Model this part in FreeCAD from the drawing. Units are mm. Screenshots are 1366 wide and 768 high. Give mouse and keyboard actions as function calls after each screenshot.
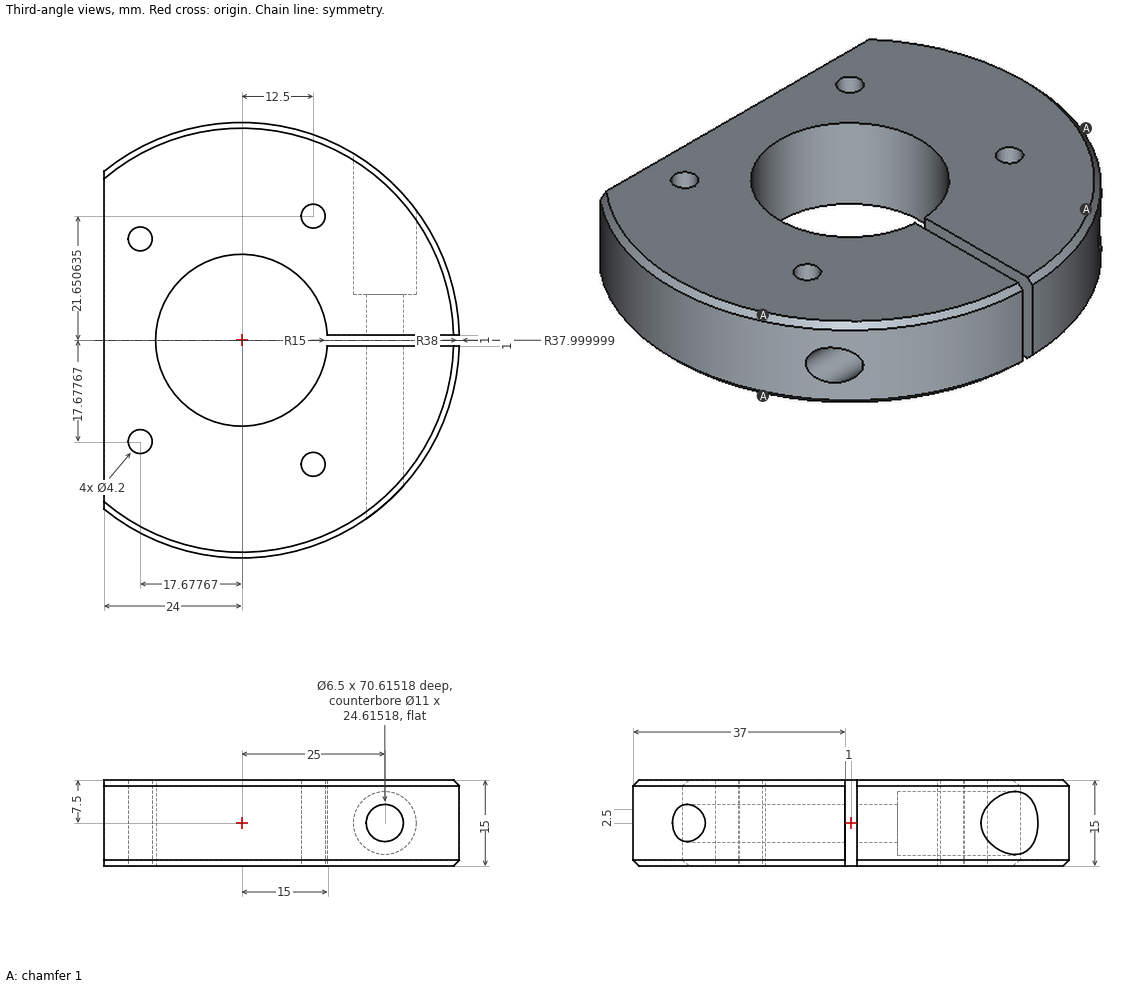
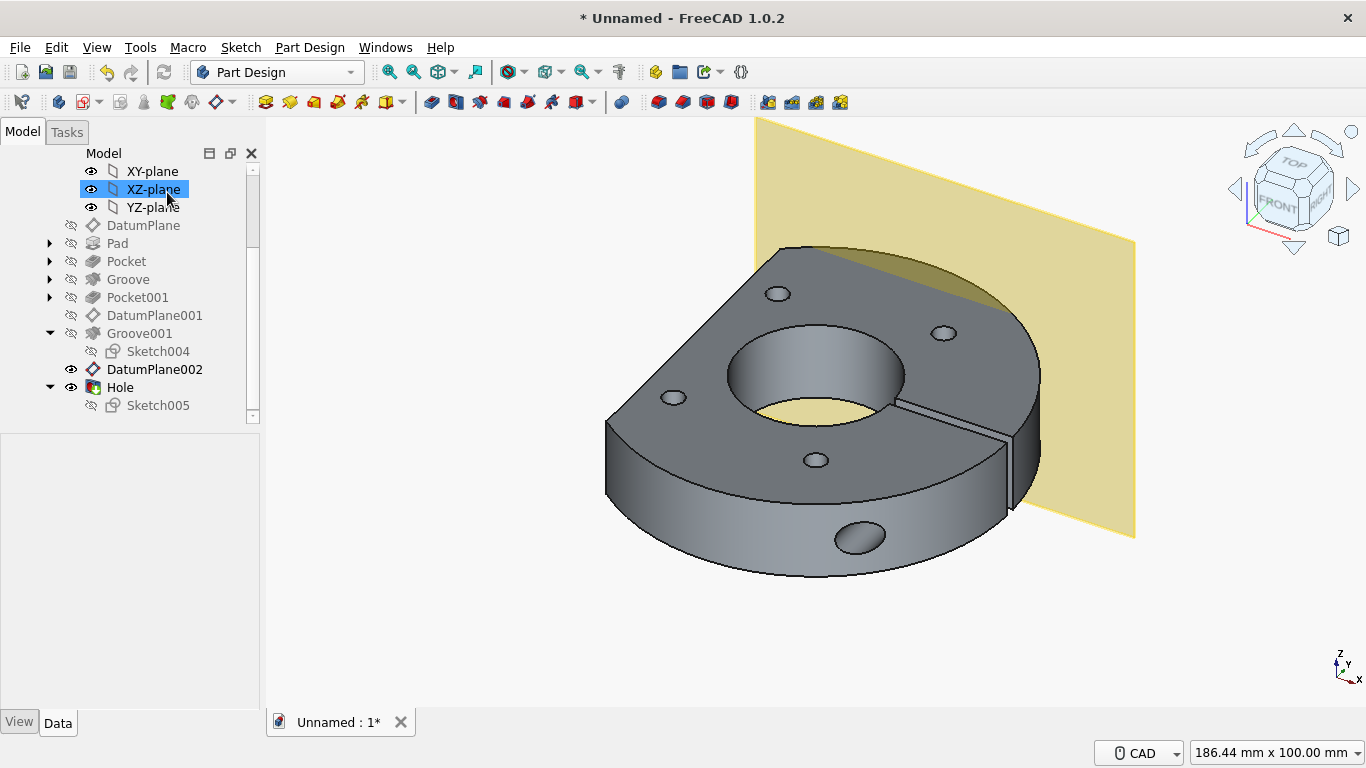
click(116, 369)
key(space)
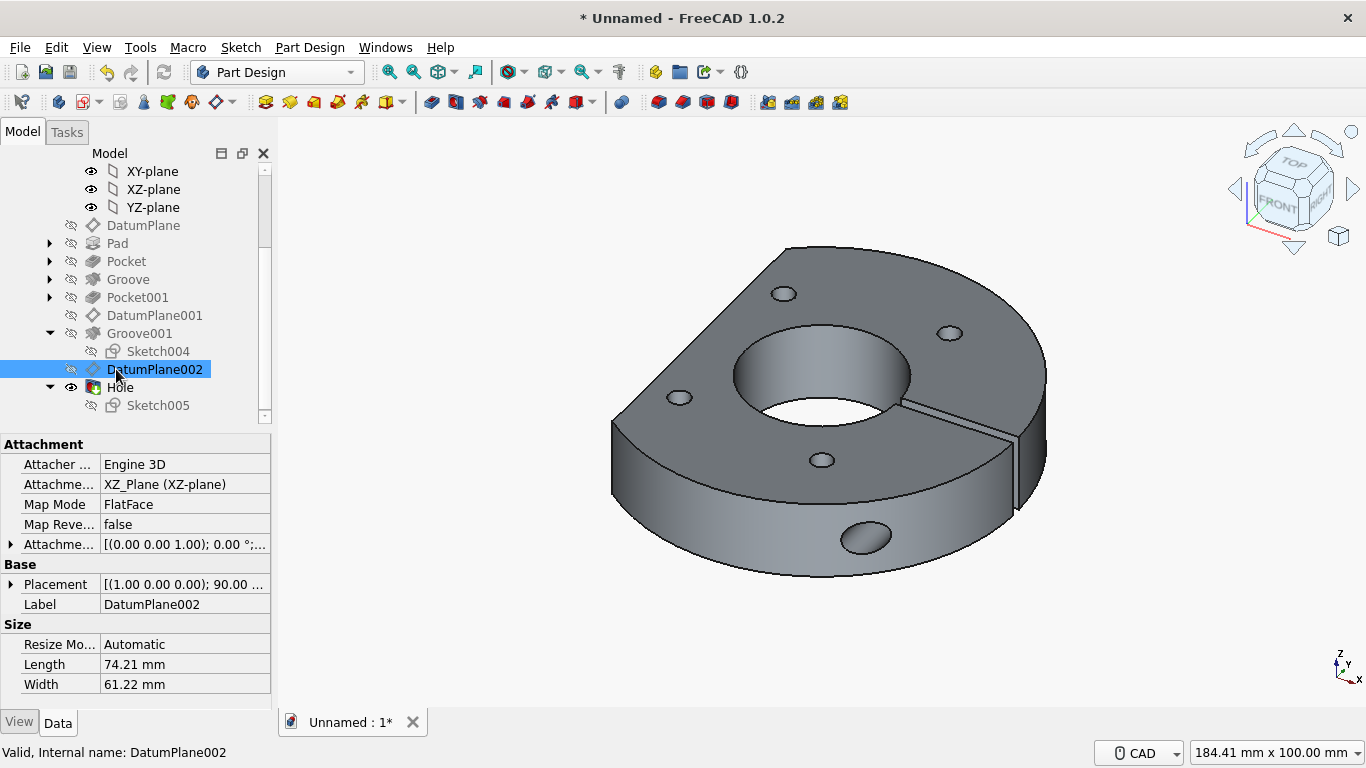
click(801, 503)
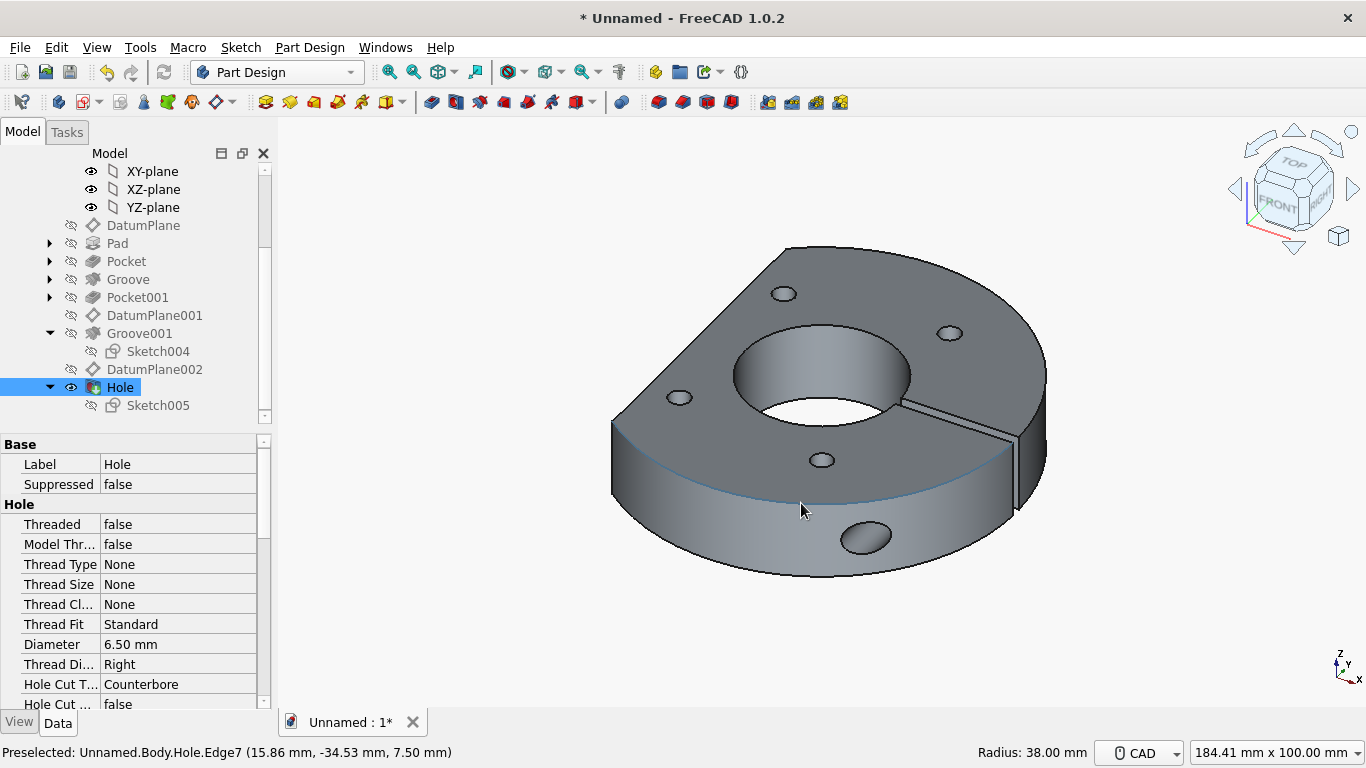
click(1046, 381, ctrl)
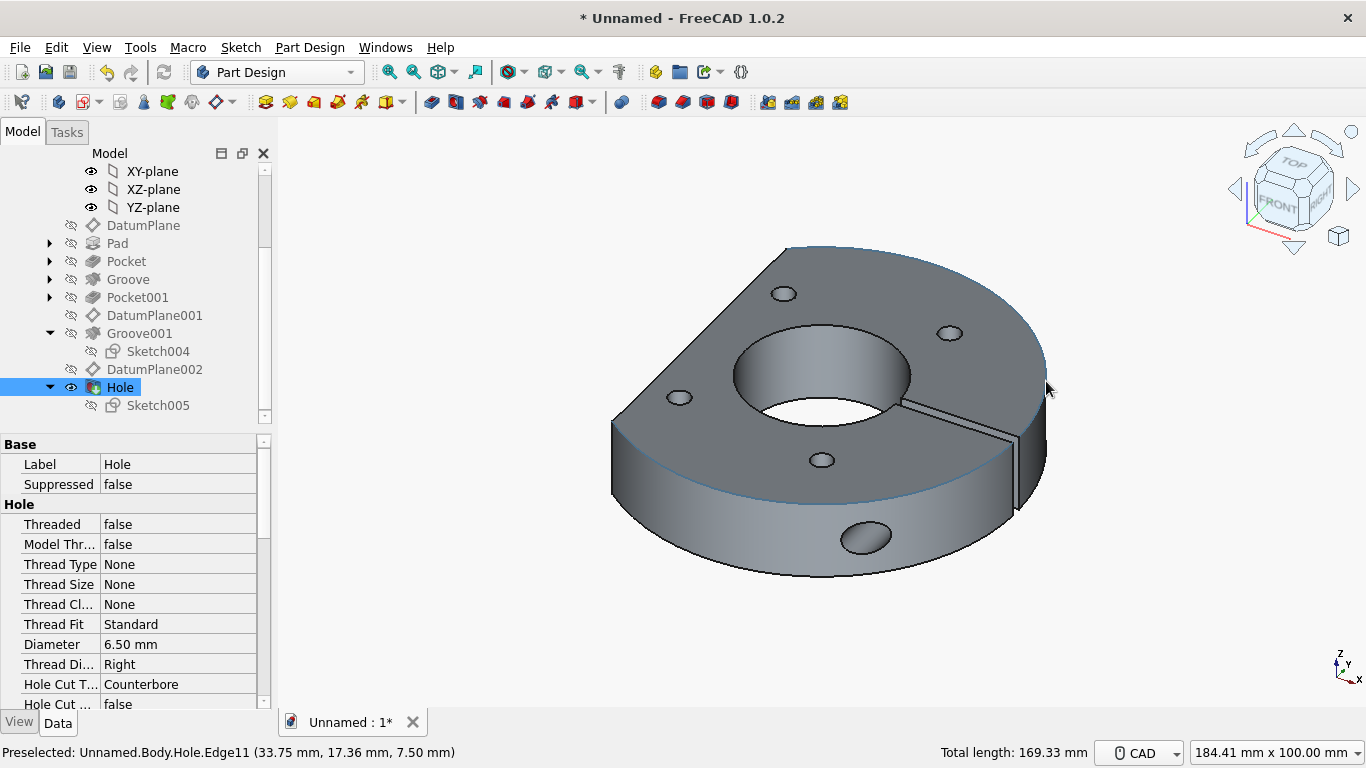
key(0)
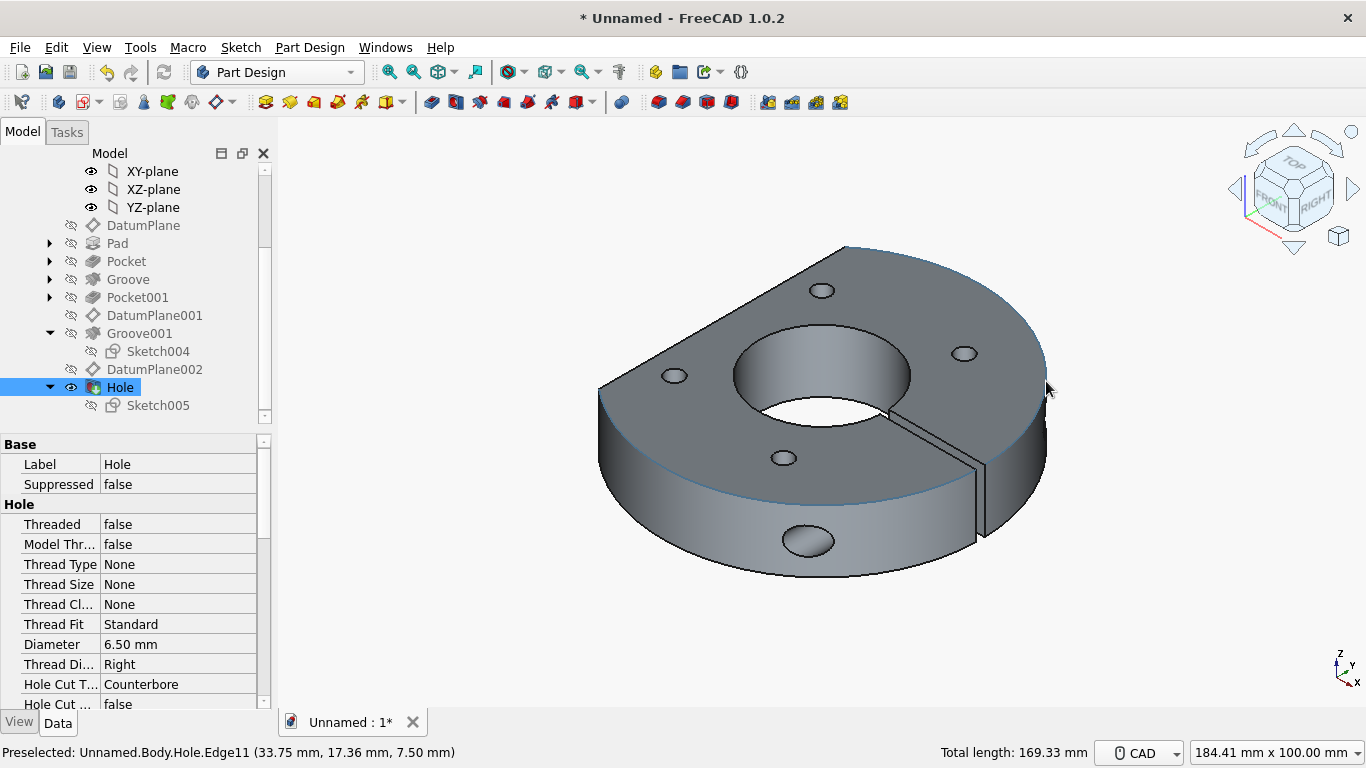
key(2)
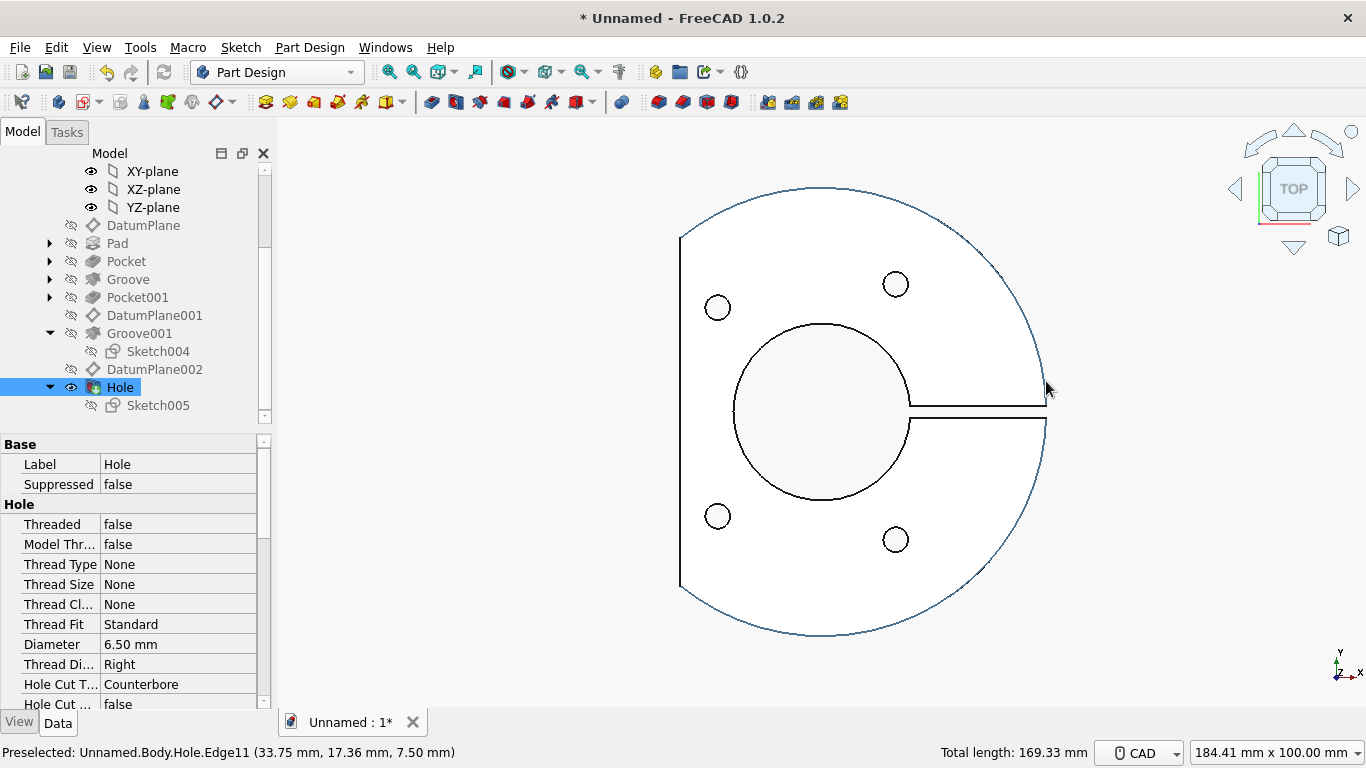
key(1)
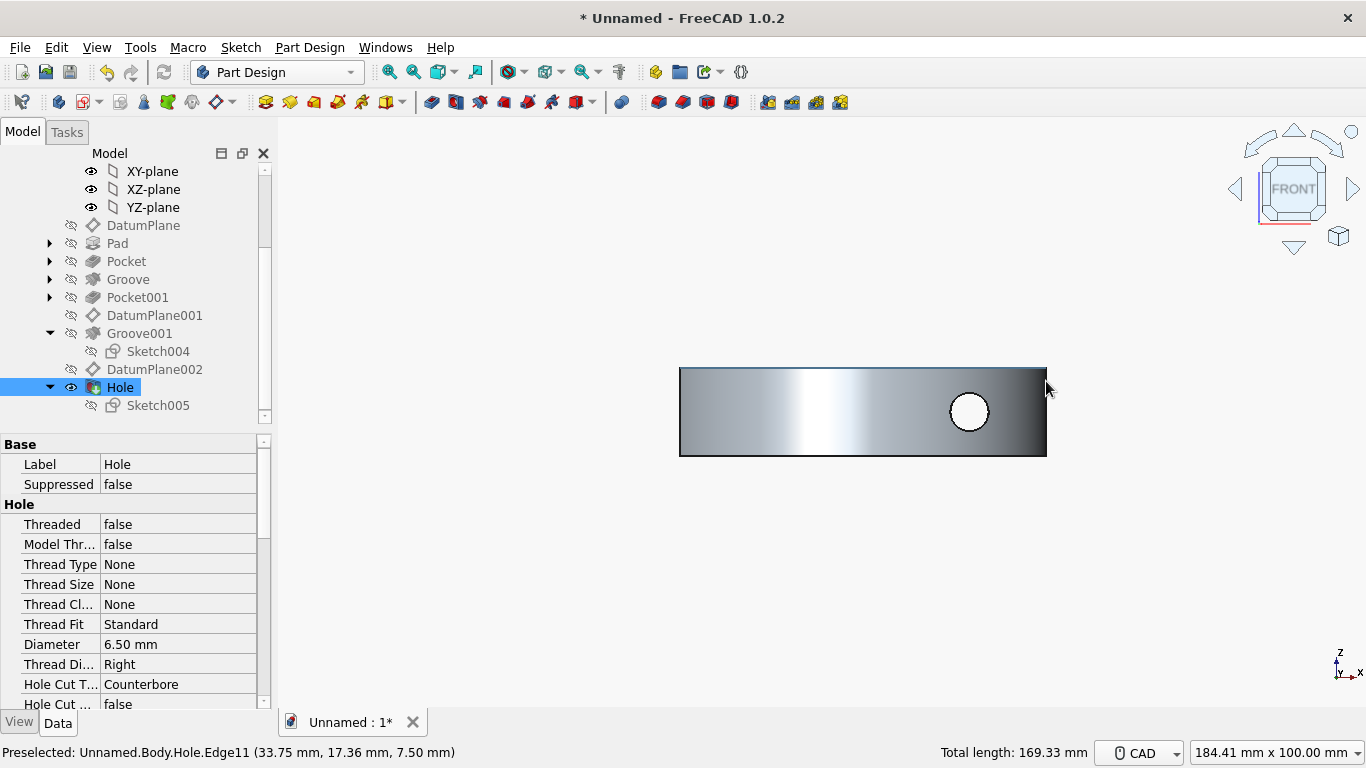
key(v)
key(f)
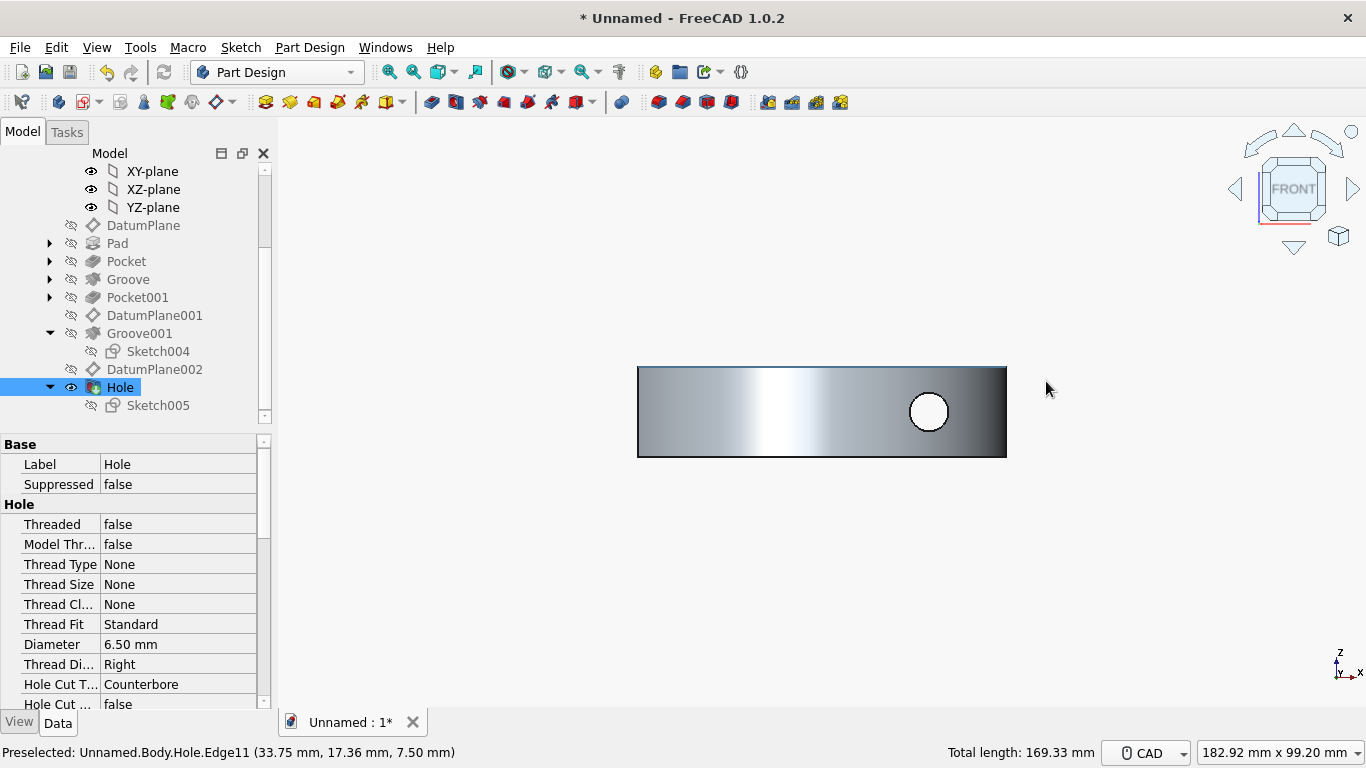
click(875, 456, ctrl)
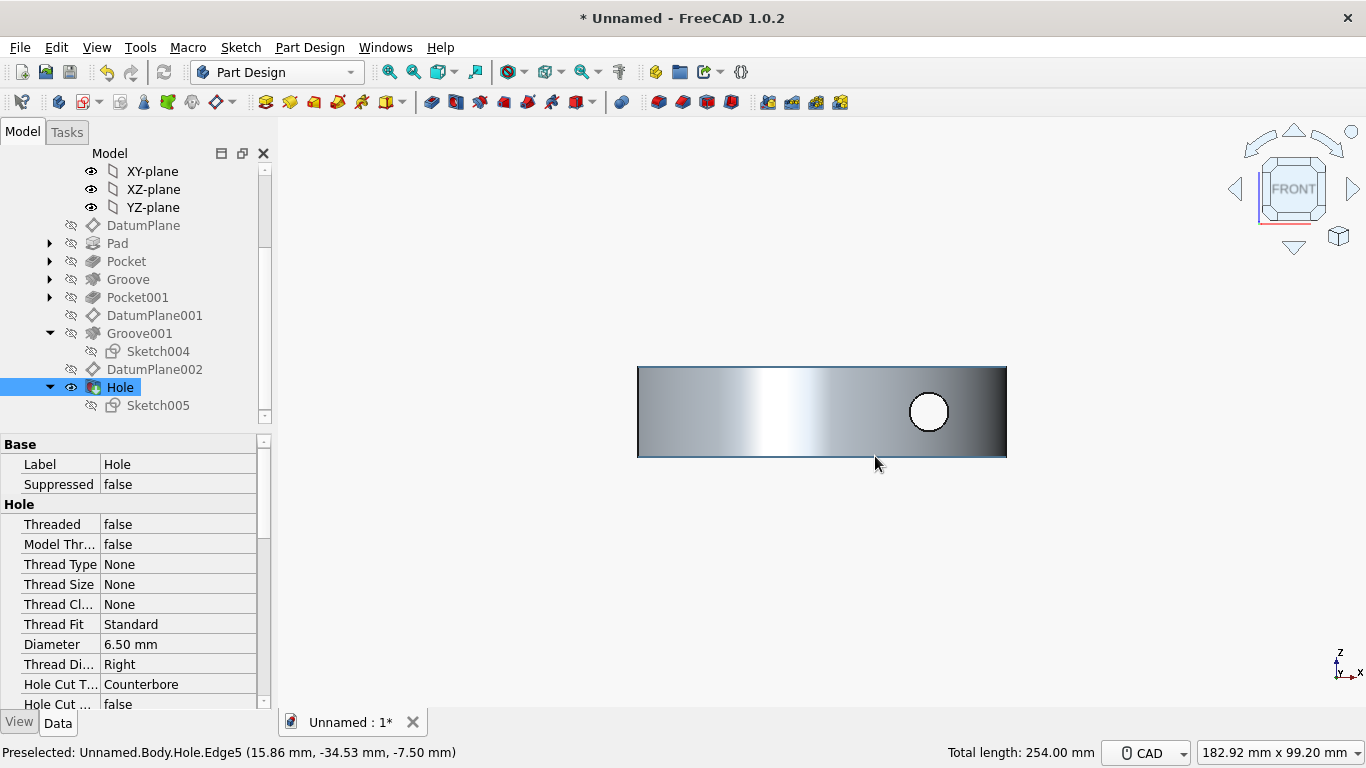
key(3)